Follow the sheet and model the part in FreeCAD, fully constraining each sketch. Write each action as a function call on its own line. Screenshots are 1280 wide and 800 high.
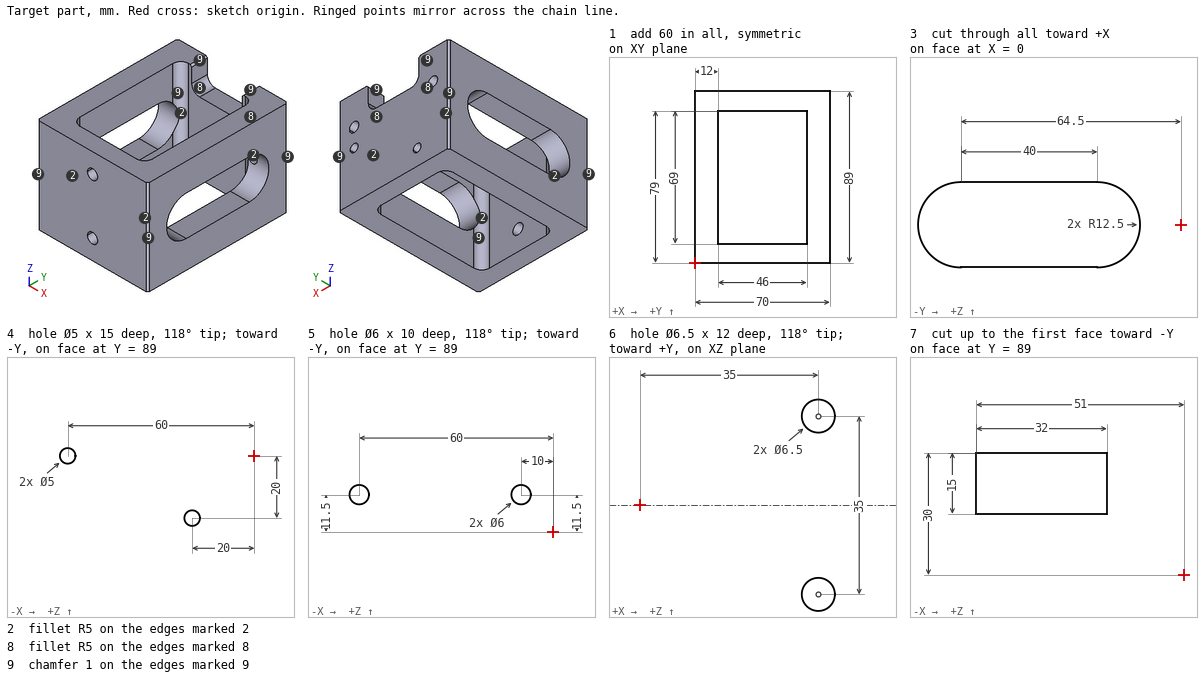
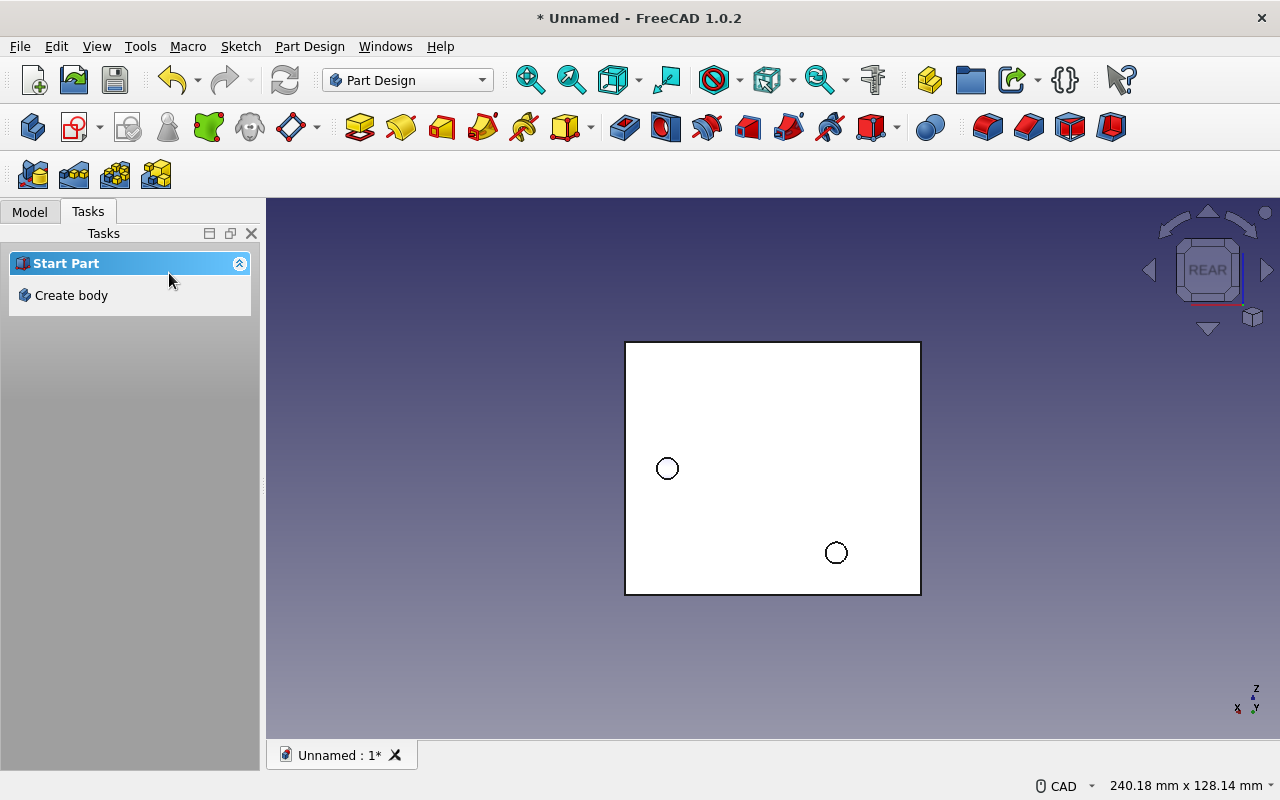
click(773, 468)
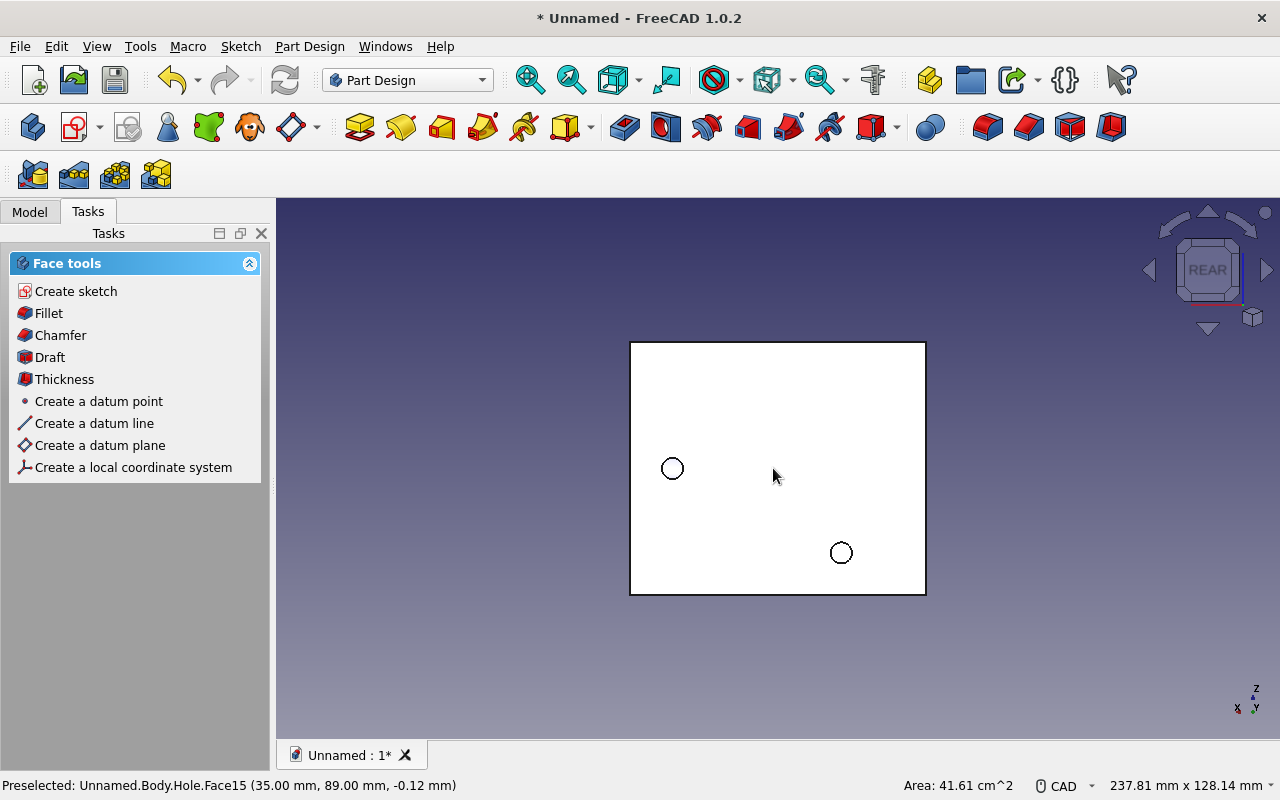
click(74, 128)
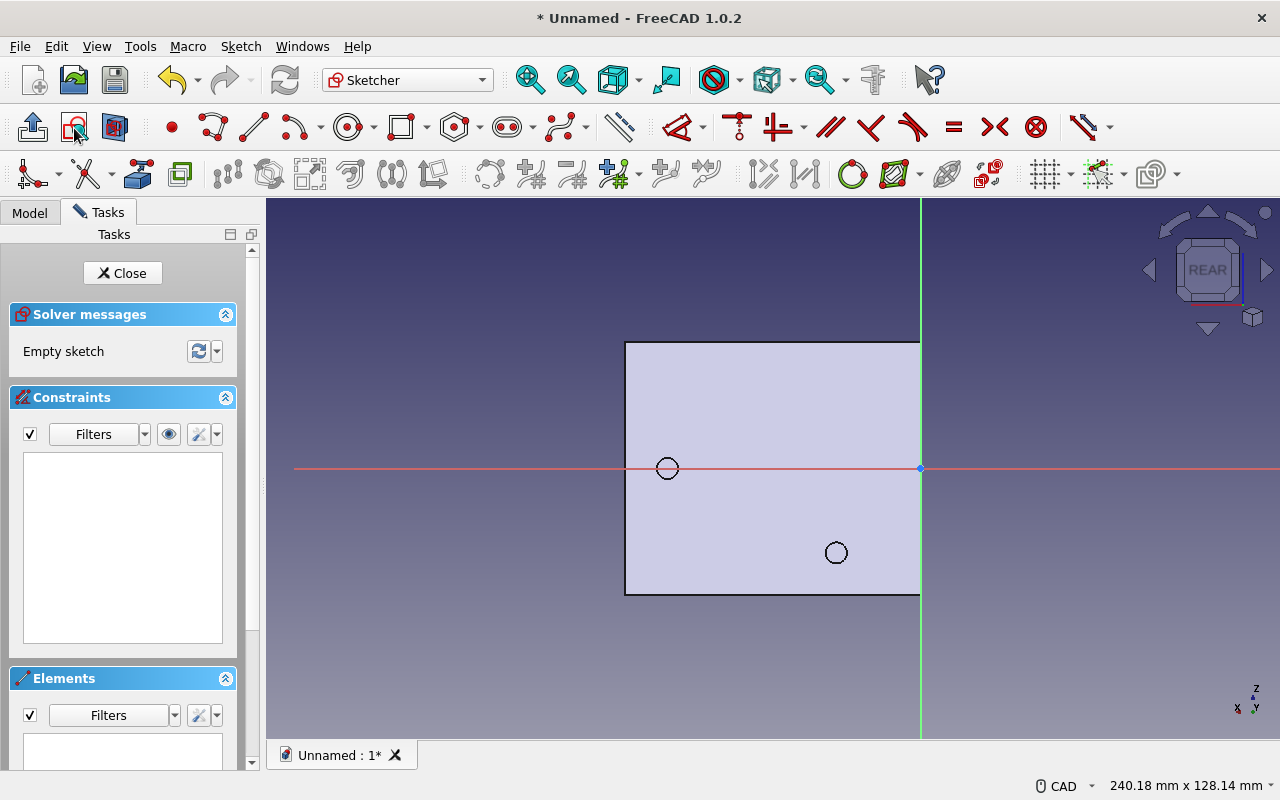
scroll(856, 413, up, 4)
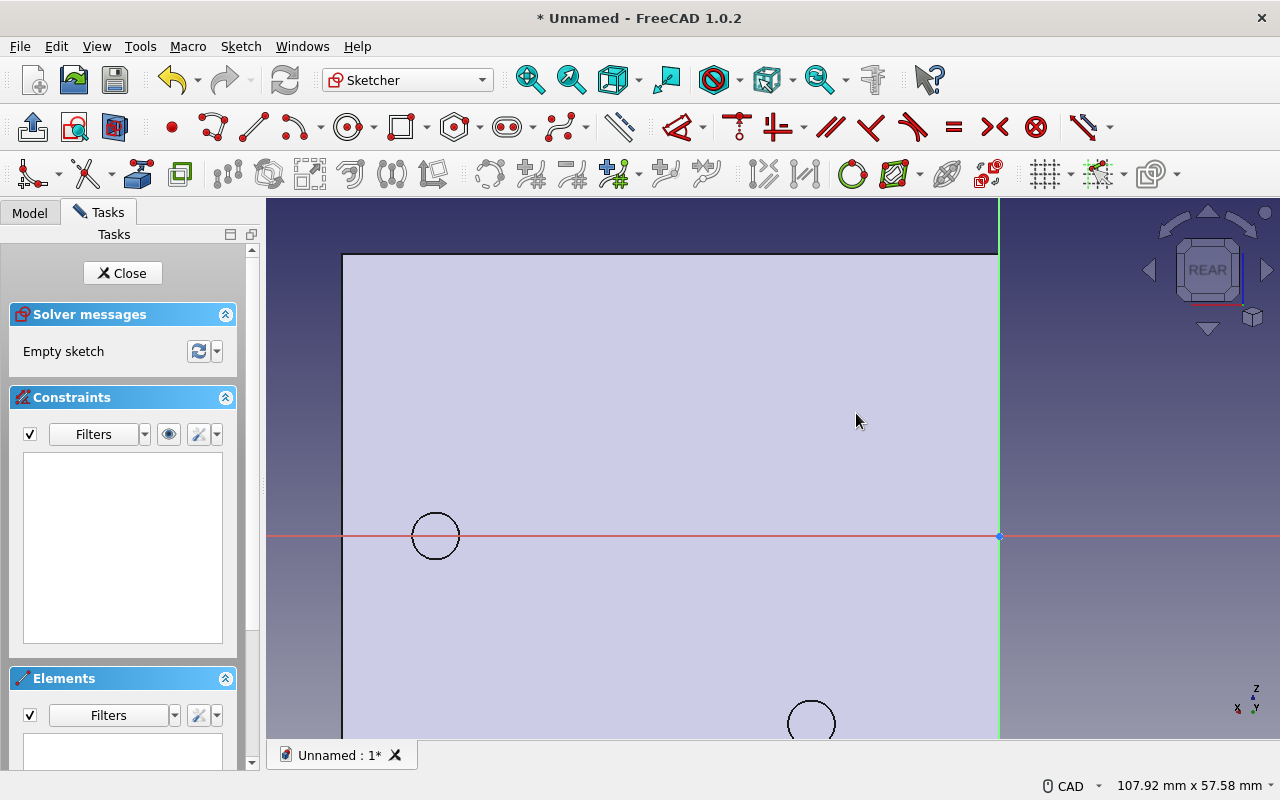
click(348, 128)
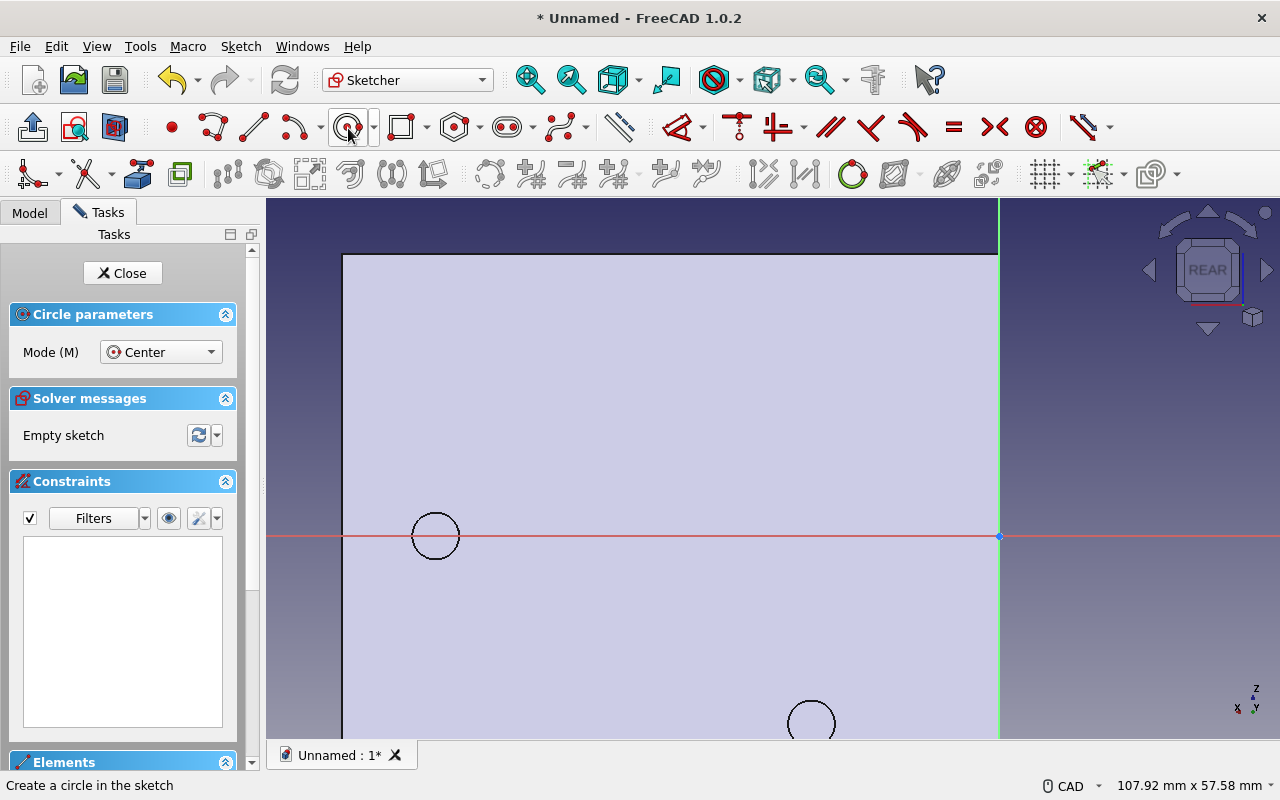
click(905, 428)
click(925, 408)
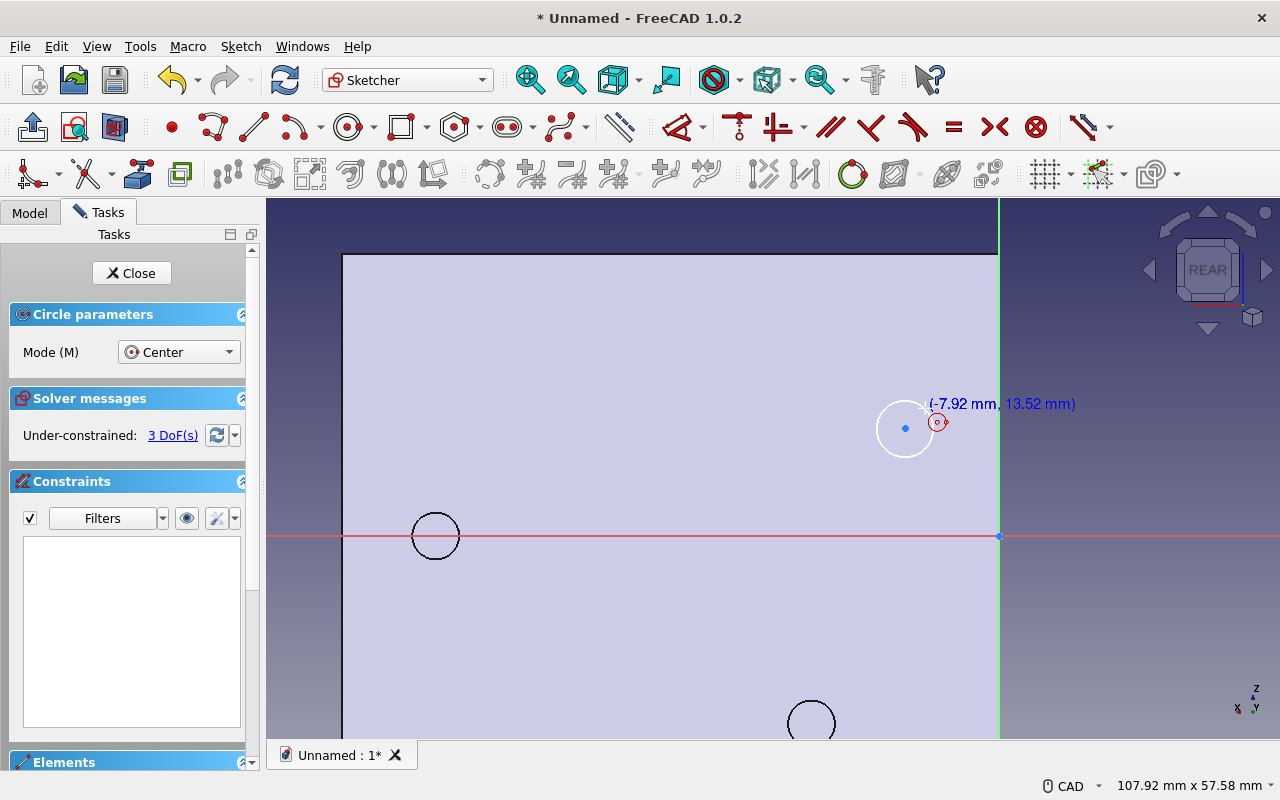
click(436, 428)
click(456, 408)
key(Escape)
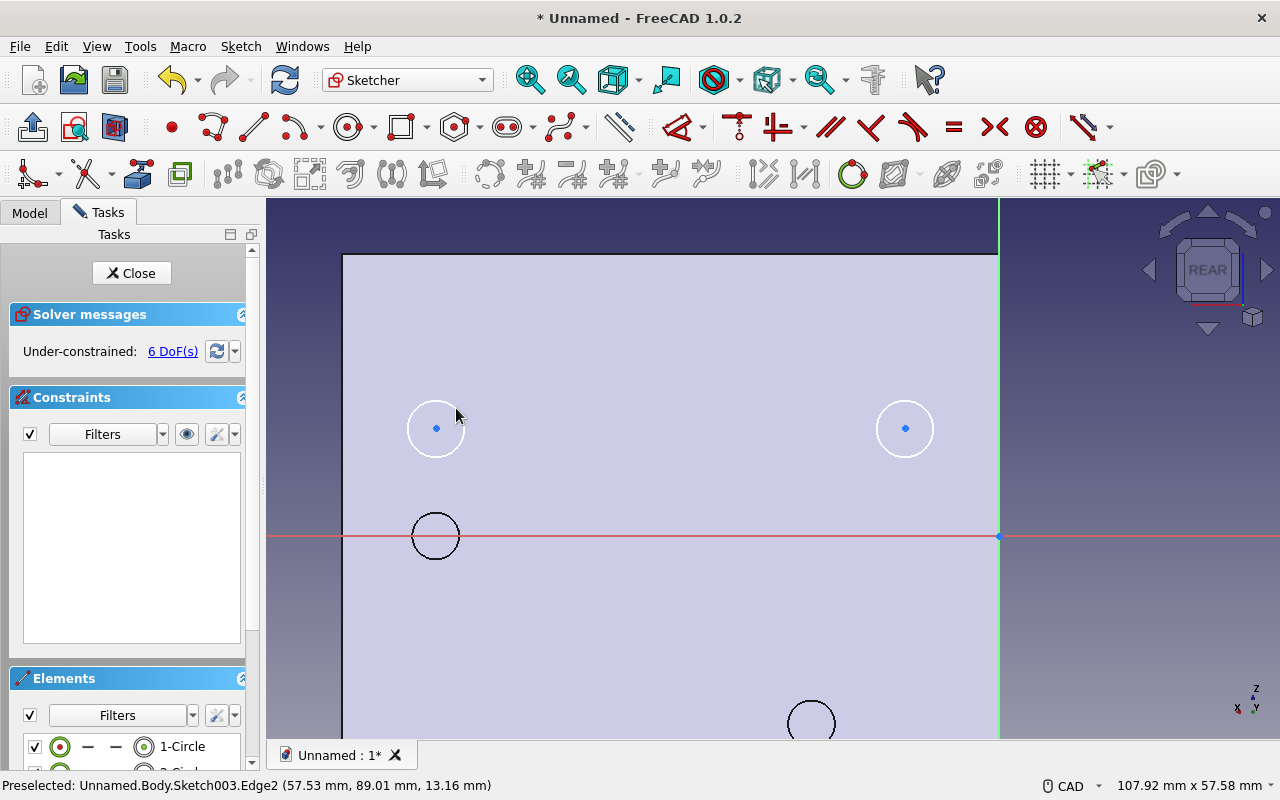
click(925, 409)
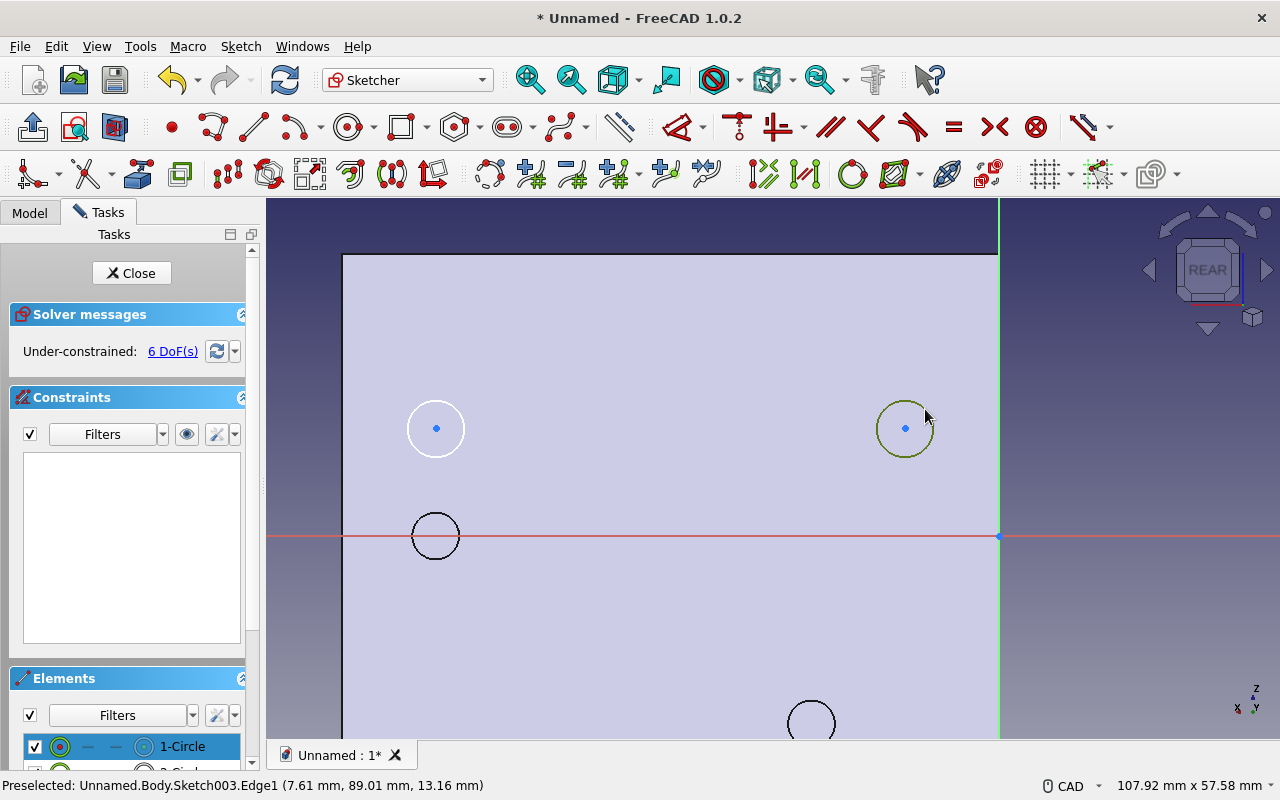
click(456, 409)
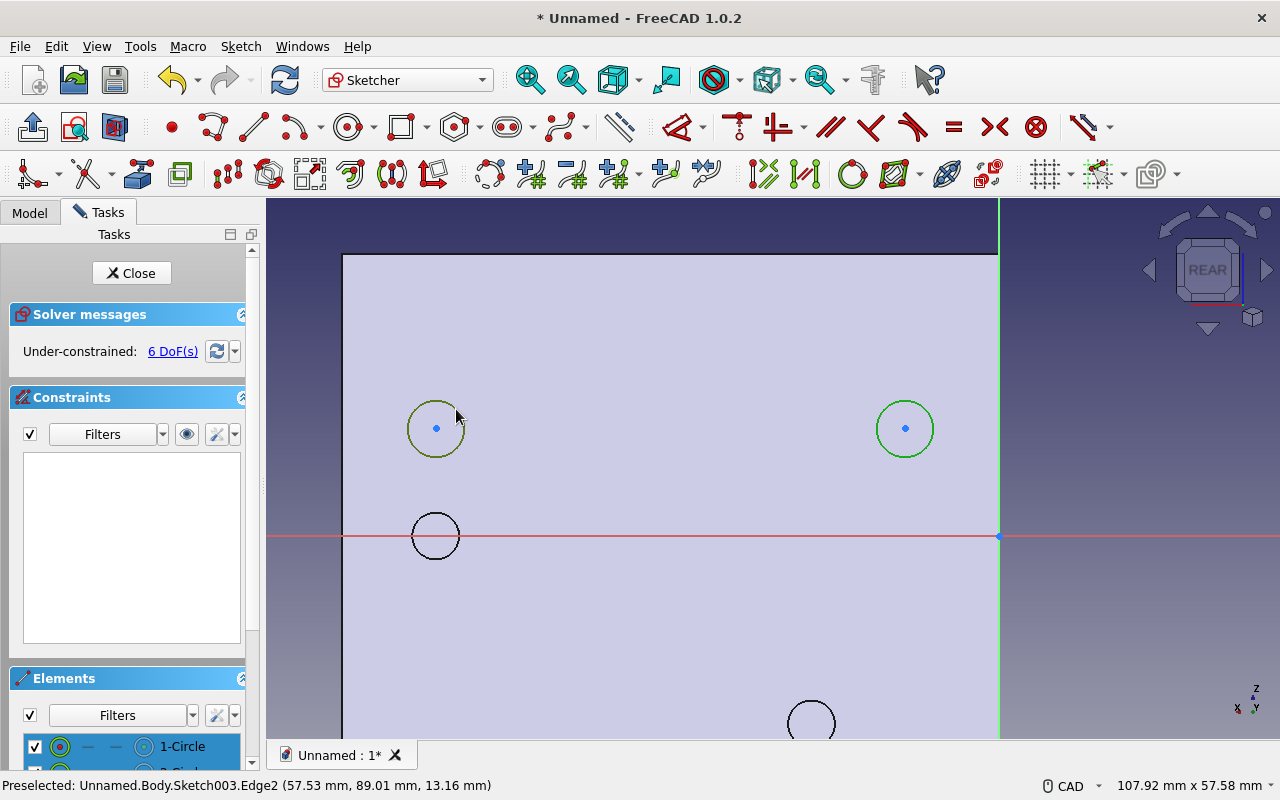
click(954, 128)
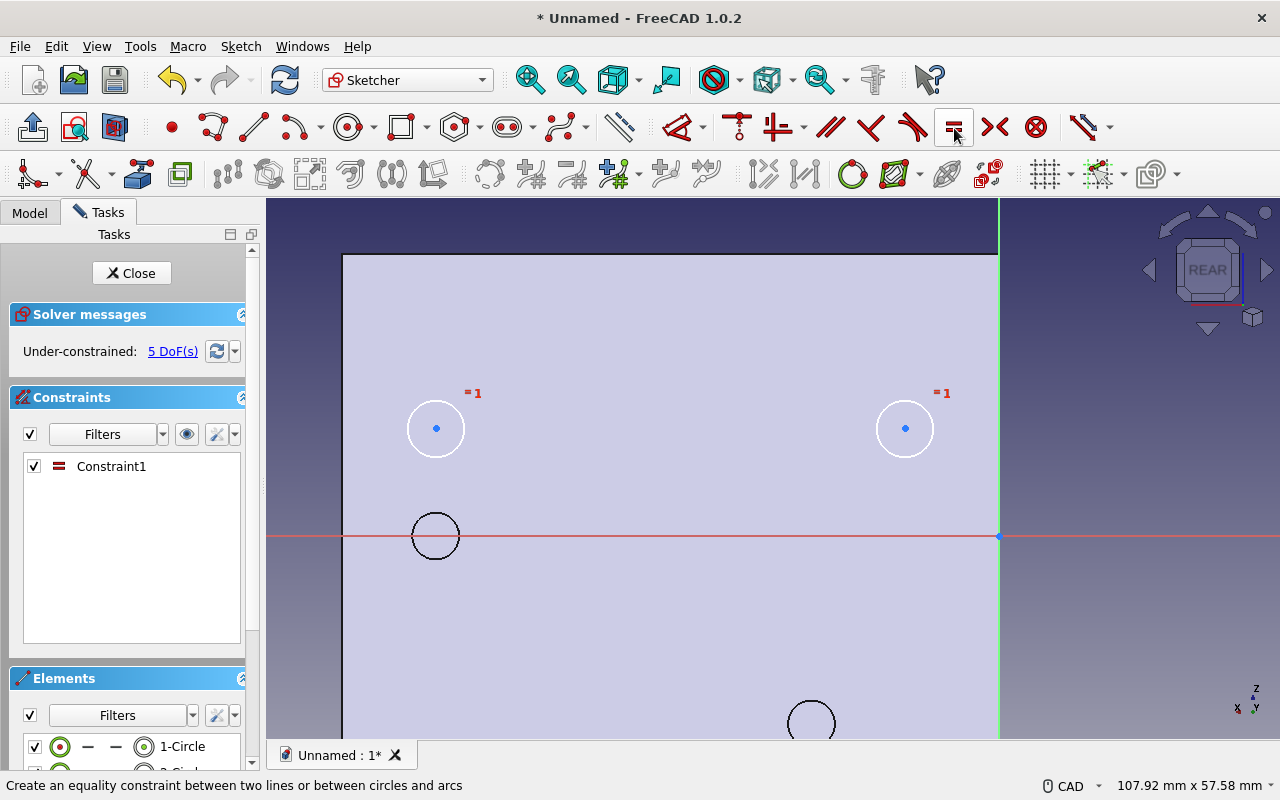
key(d)